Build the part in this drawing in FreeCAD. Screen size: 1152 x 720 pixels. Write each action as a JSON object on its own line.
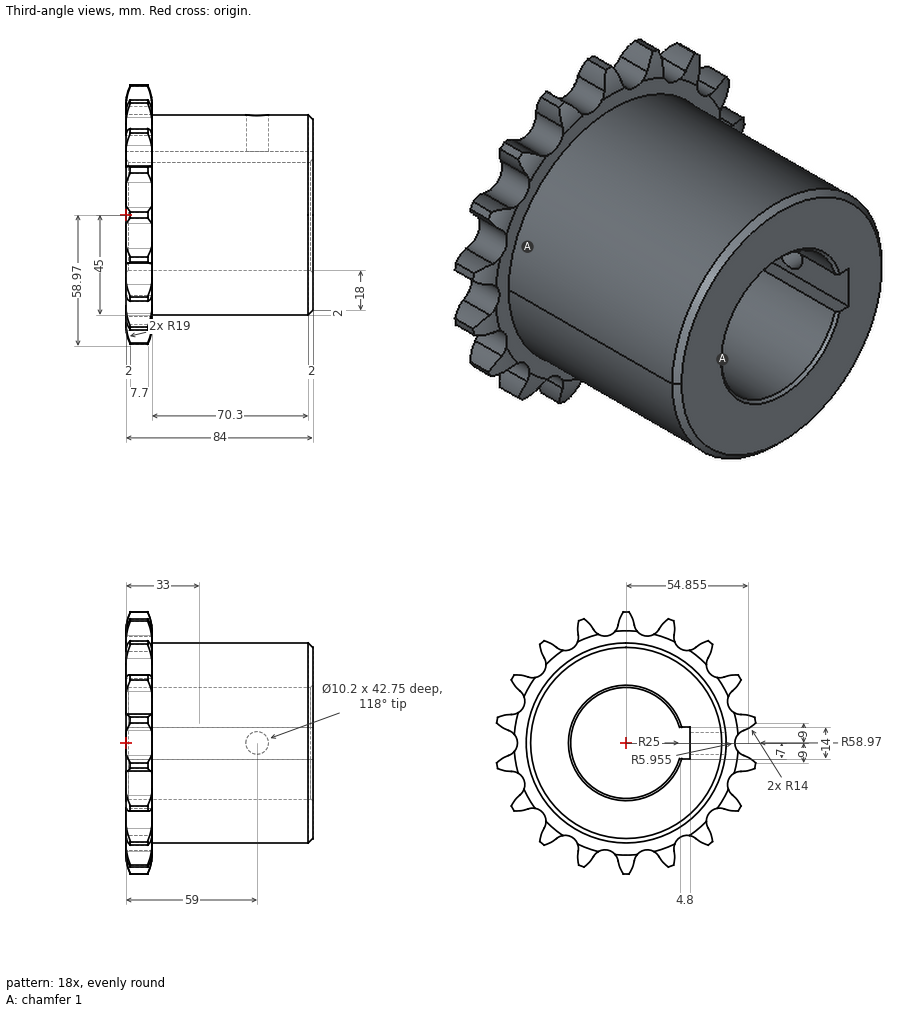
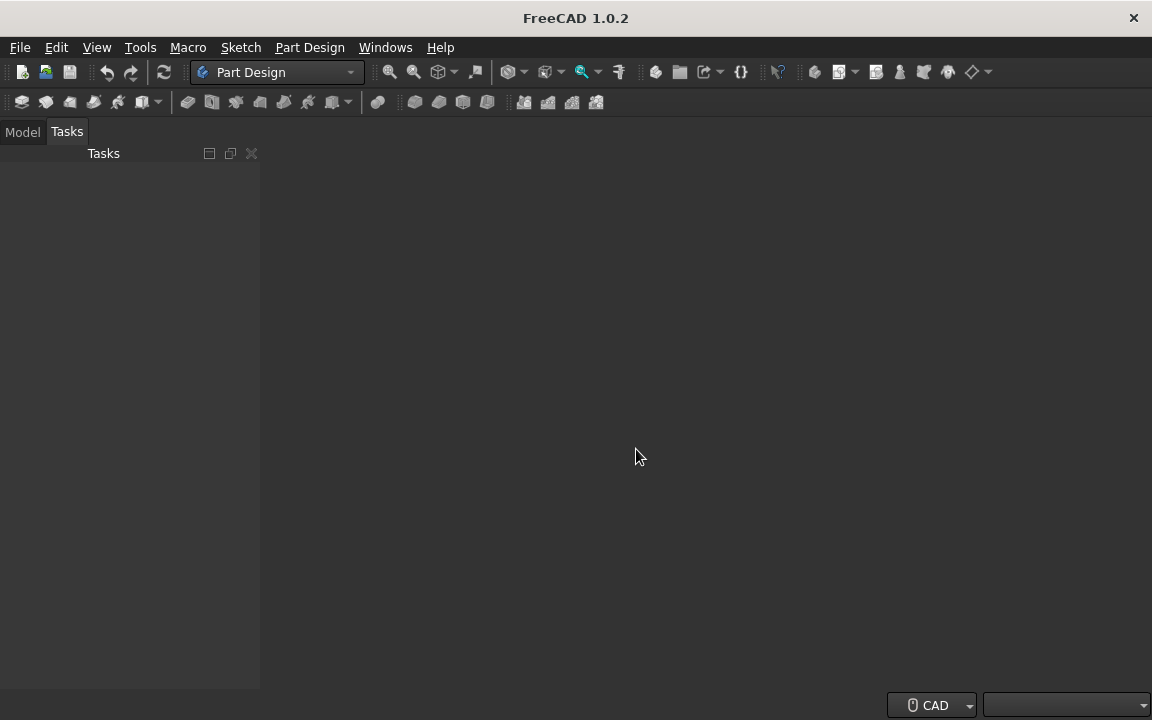
{"action": "left_click", "coordinate": [22, 72]}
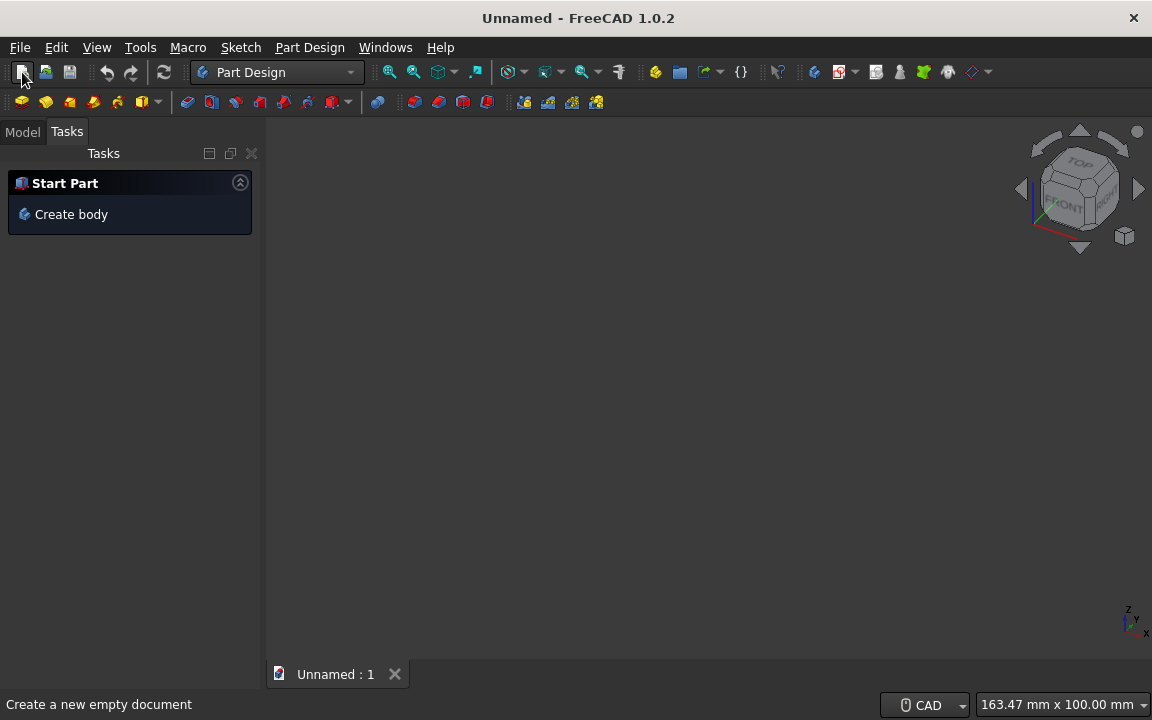
{"action": "left_click", "coordinate": [840, 72]}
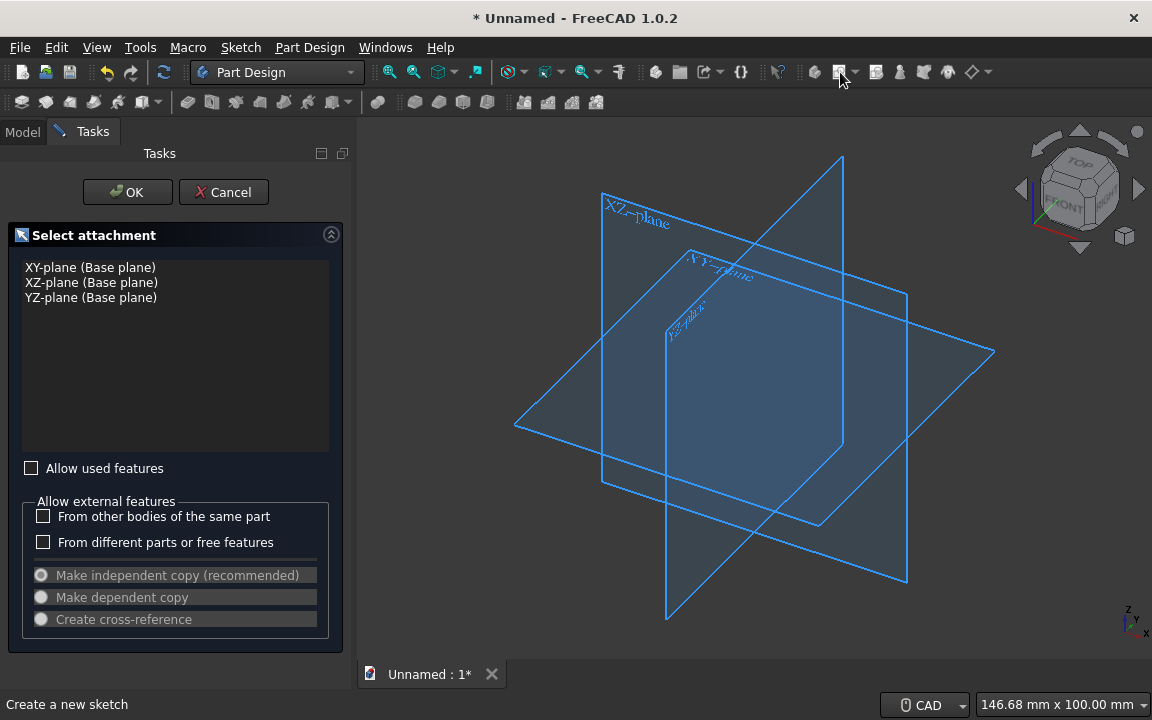
{"action": "left_click", "coordinate": [82, 268]}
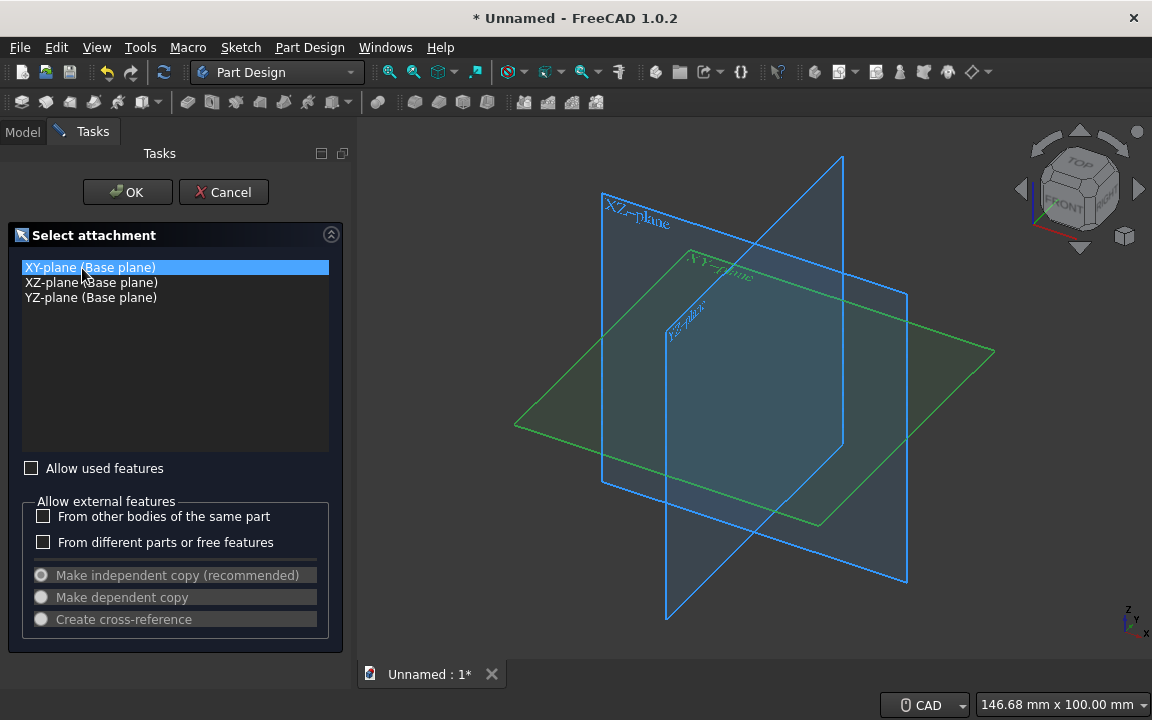
{"action": "left_click", "coordinate": [128, 192]}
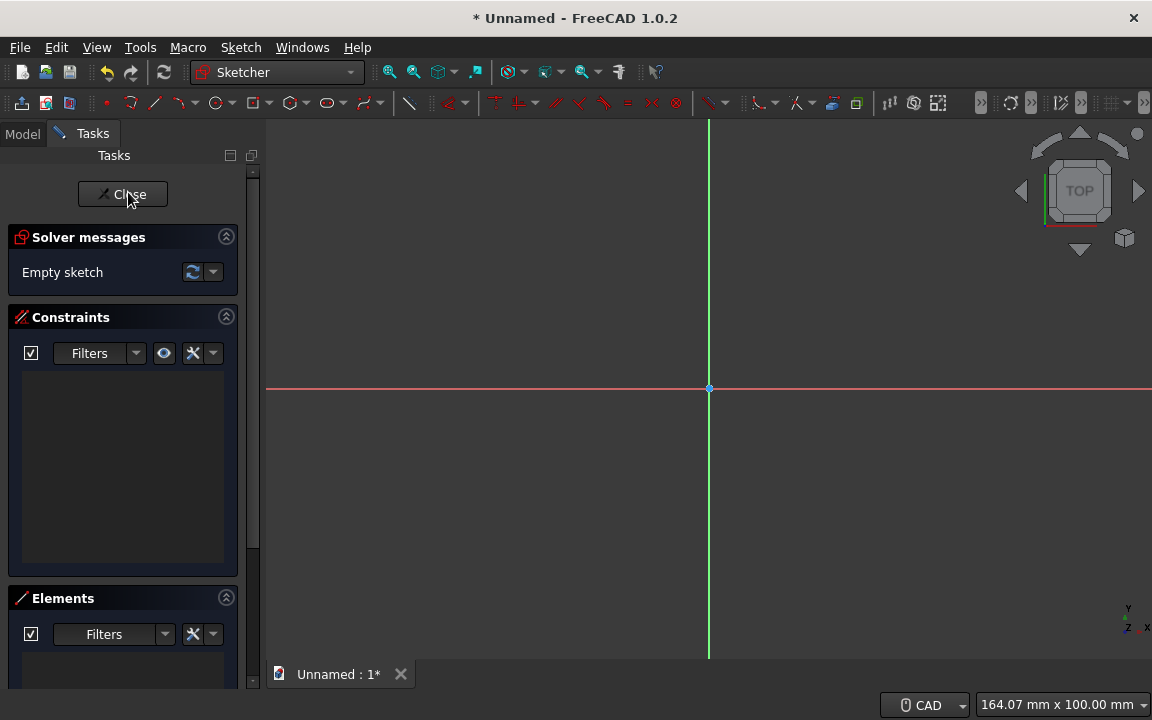
{"action": "scroll", "coordinate": [294, 147], "scroll_direction": "down", "scroll_amount": 2}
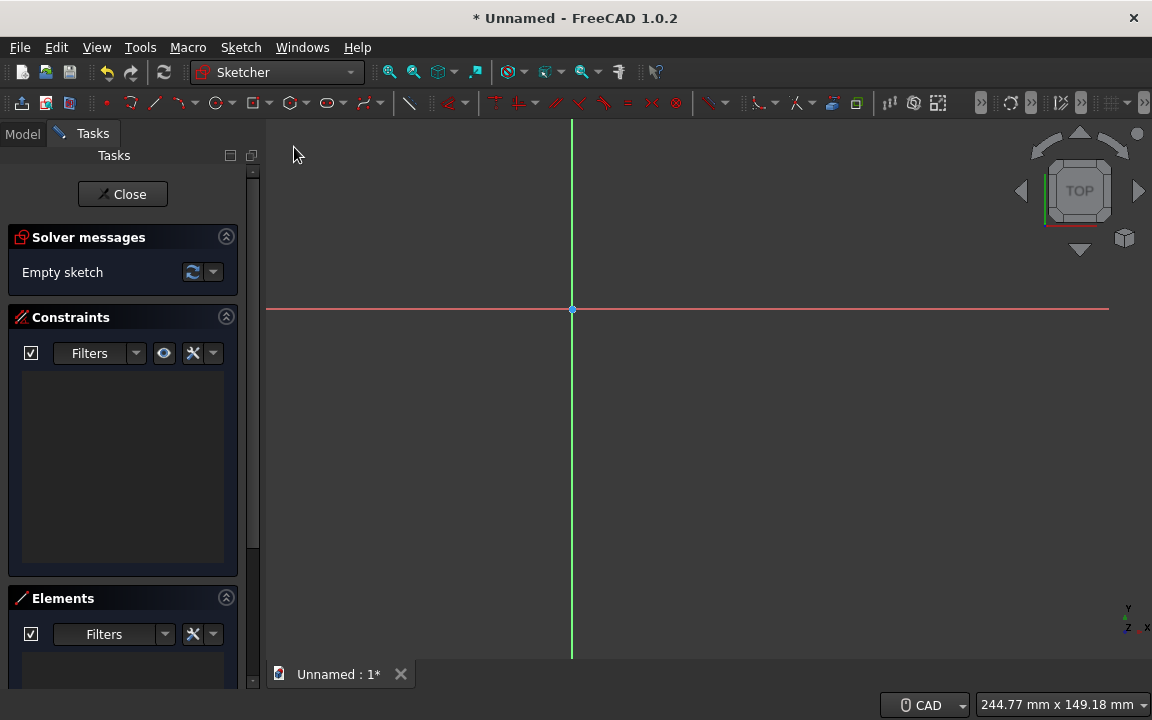
{"action": "scroll", "coordinate": [894, 471], "scroll_direction": "up", "scroll_amount": 2}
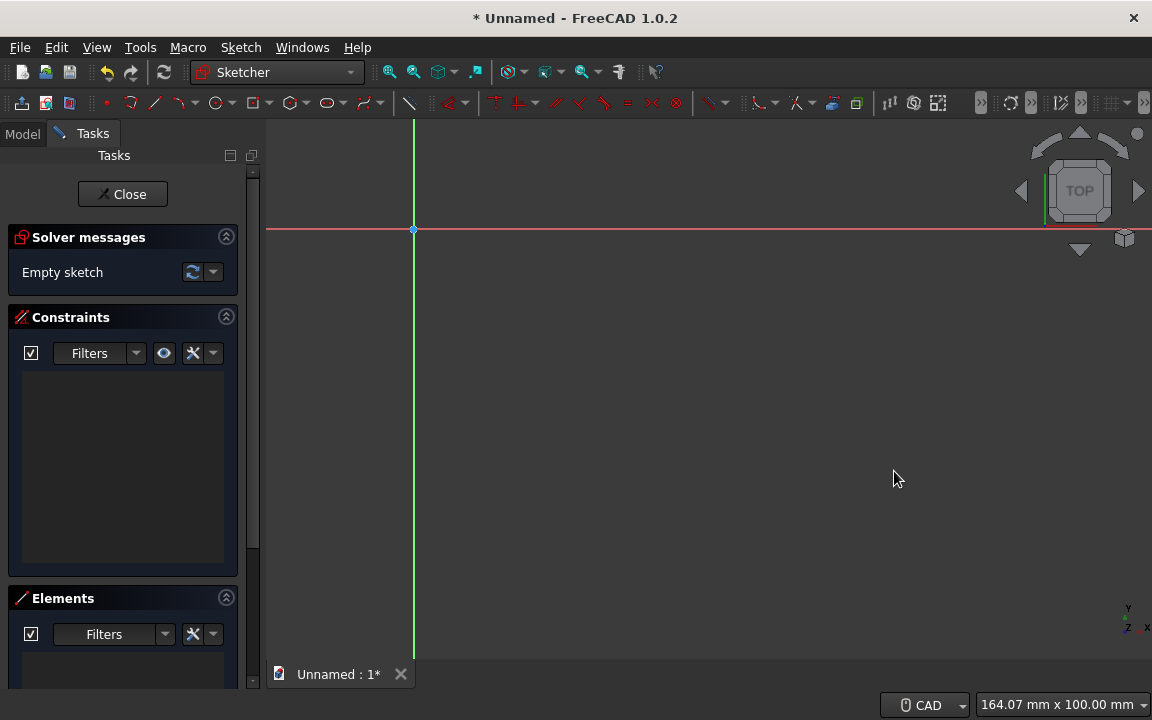
{"action": "left_click", "coordinate": [156, 104]}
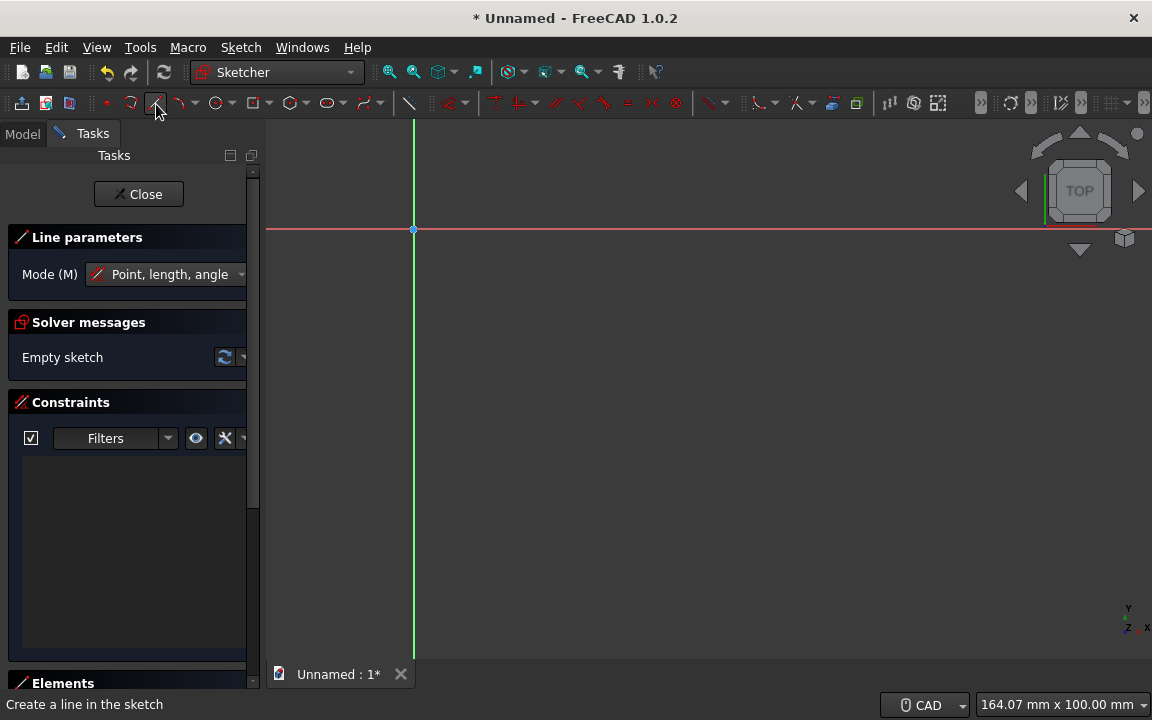
{"action": "scroll", "coordinate": [424, 548], "scroll_direction": "up", "scroll_amount": 2}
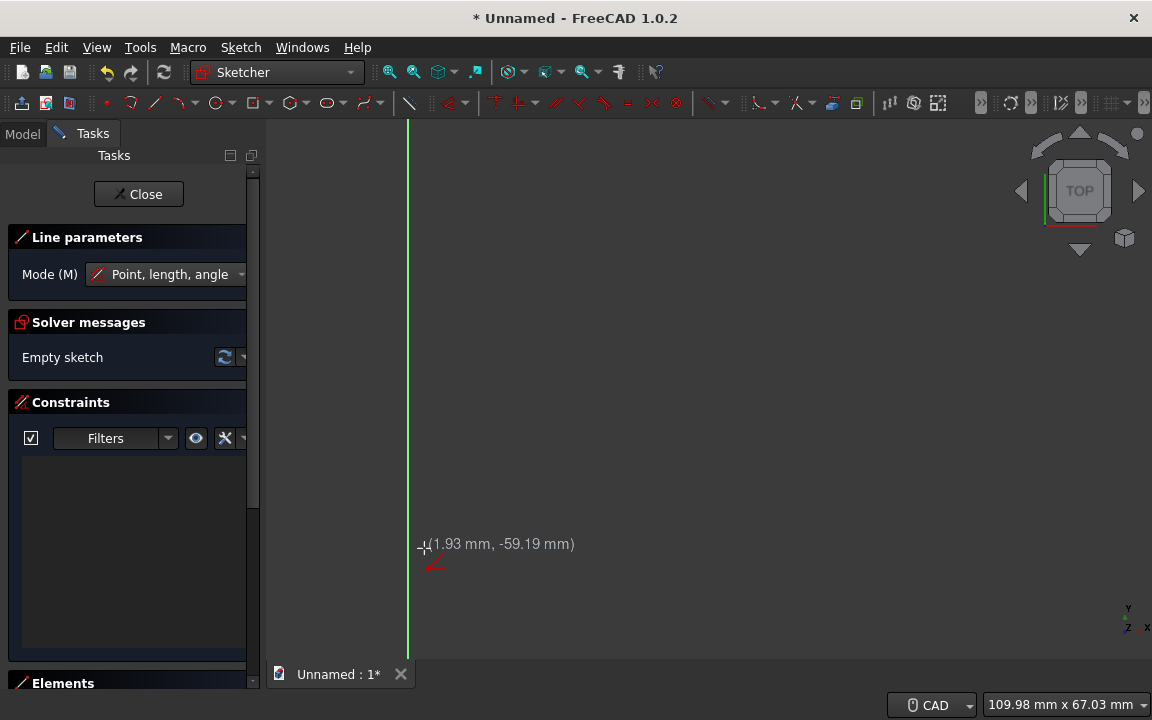
{"action": "left_click", "coordinate": [424, 547]}
{"action": "left_click", "coordinate": [486, 547]}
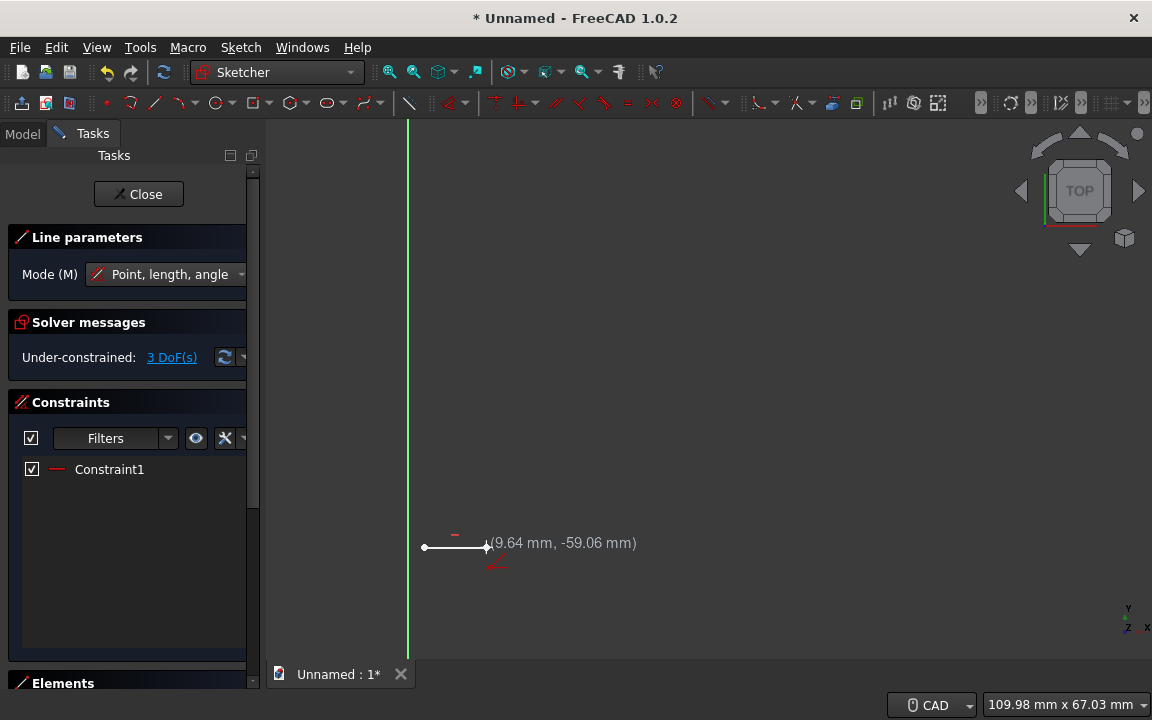
{"action": "key", "text": "g m"}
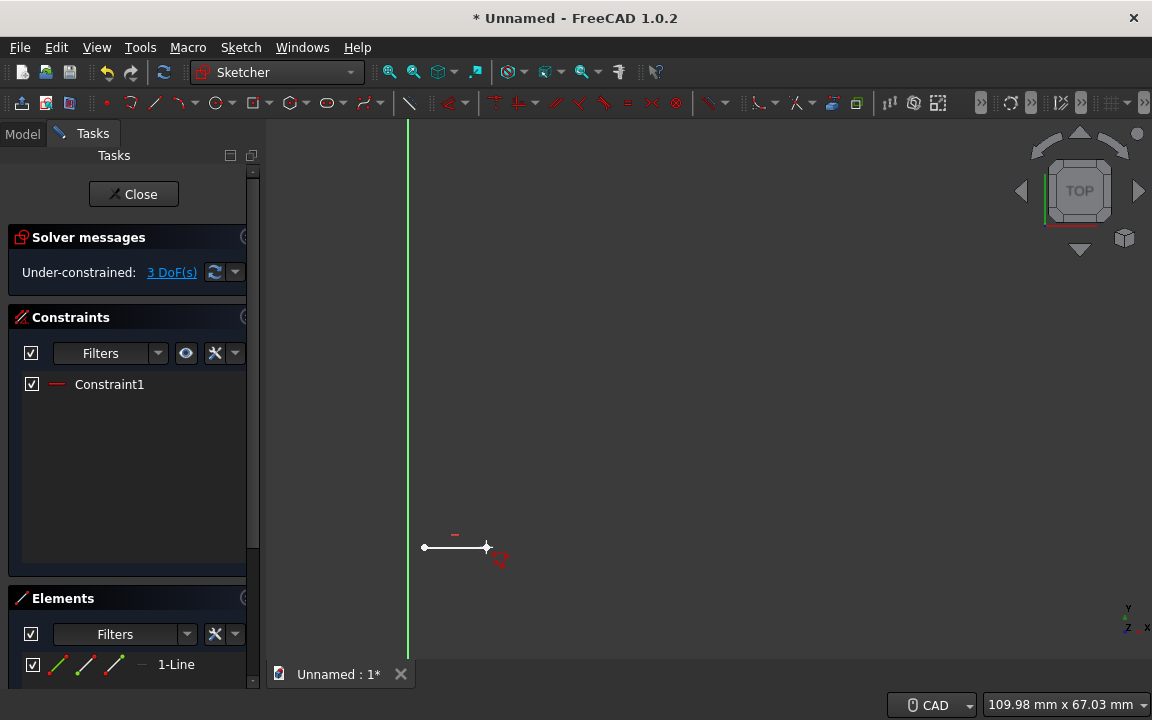
{"action": "left_click", "coordinate": [503, 479]}
{"action": "left_click", "coordinate": [503, 435]}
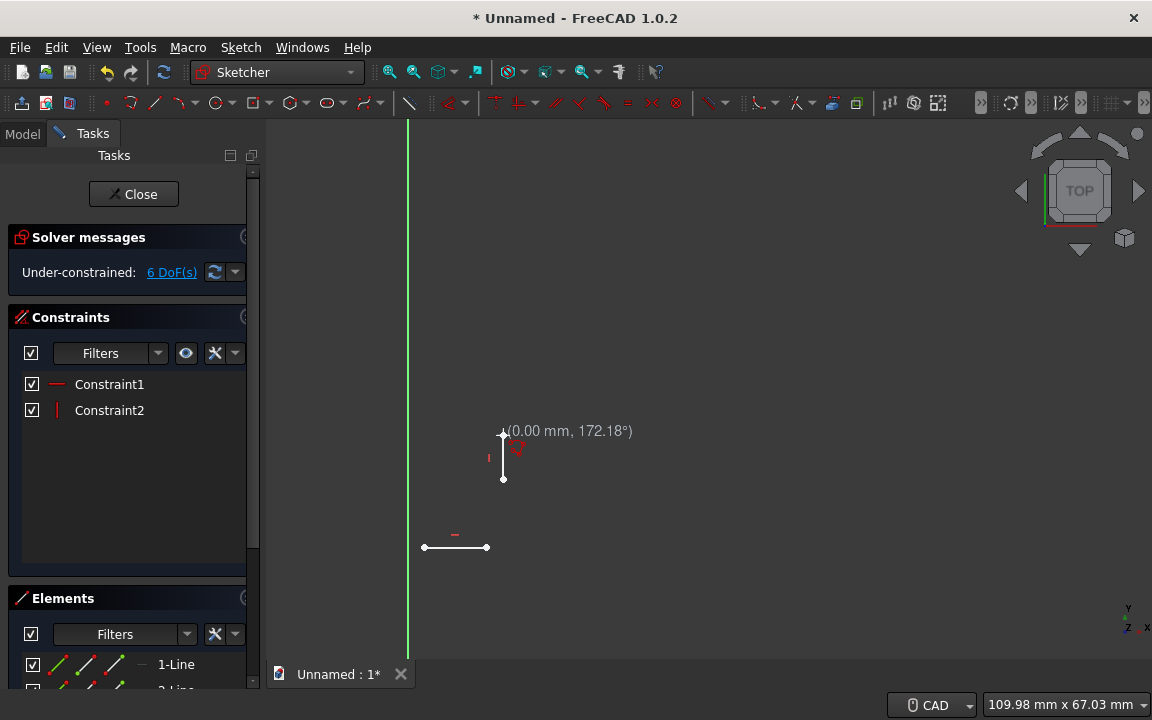
{"action": "scroll", "coordinate": [425, 550], "scroll_direction": "down", "scroll_amount": 2}